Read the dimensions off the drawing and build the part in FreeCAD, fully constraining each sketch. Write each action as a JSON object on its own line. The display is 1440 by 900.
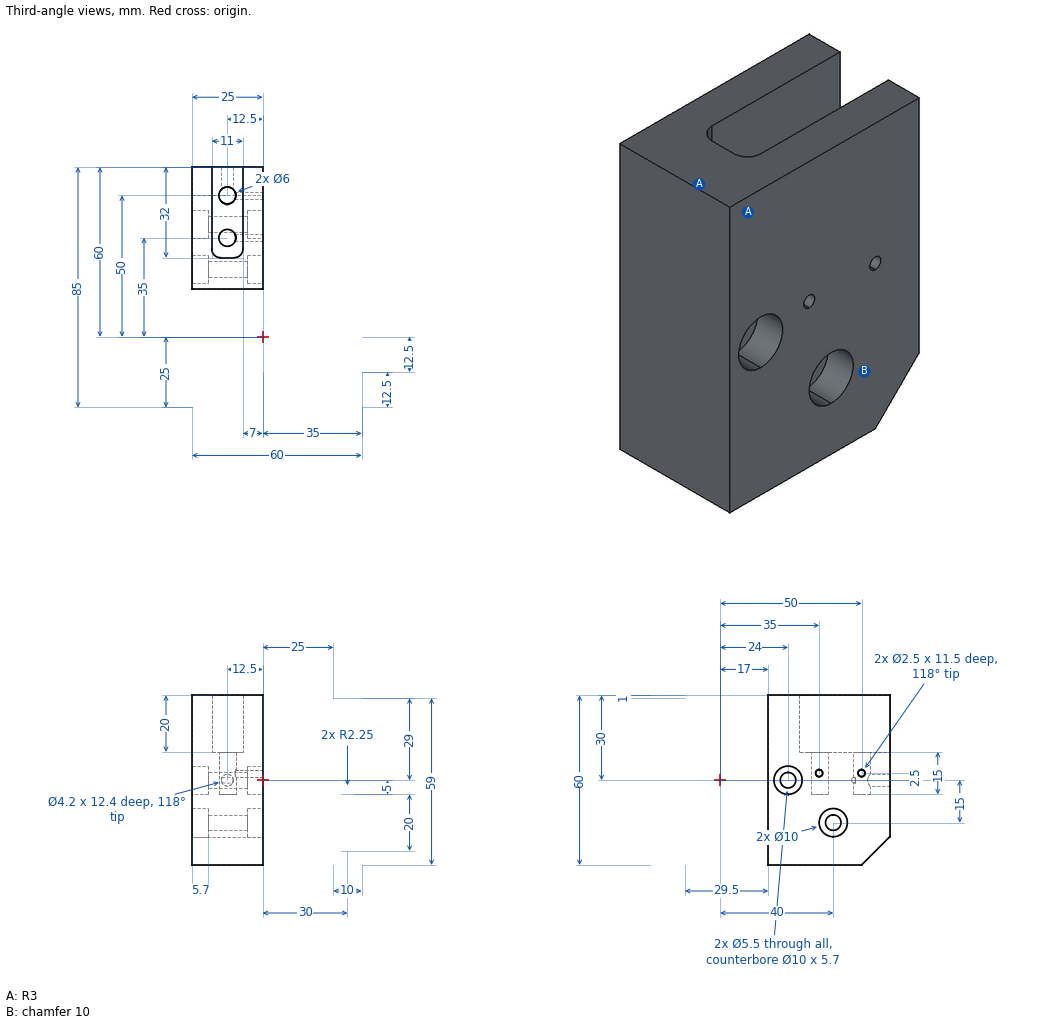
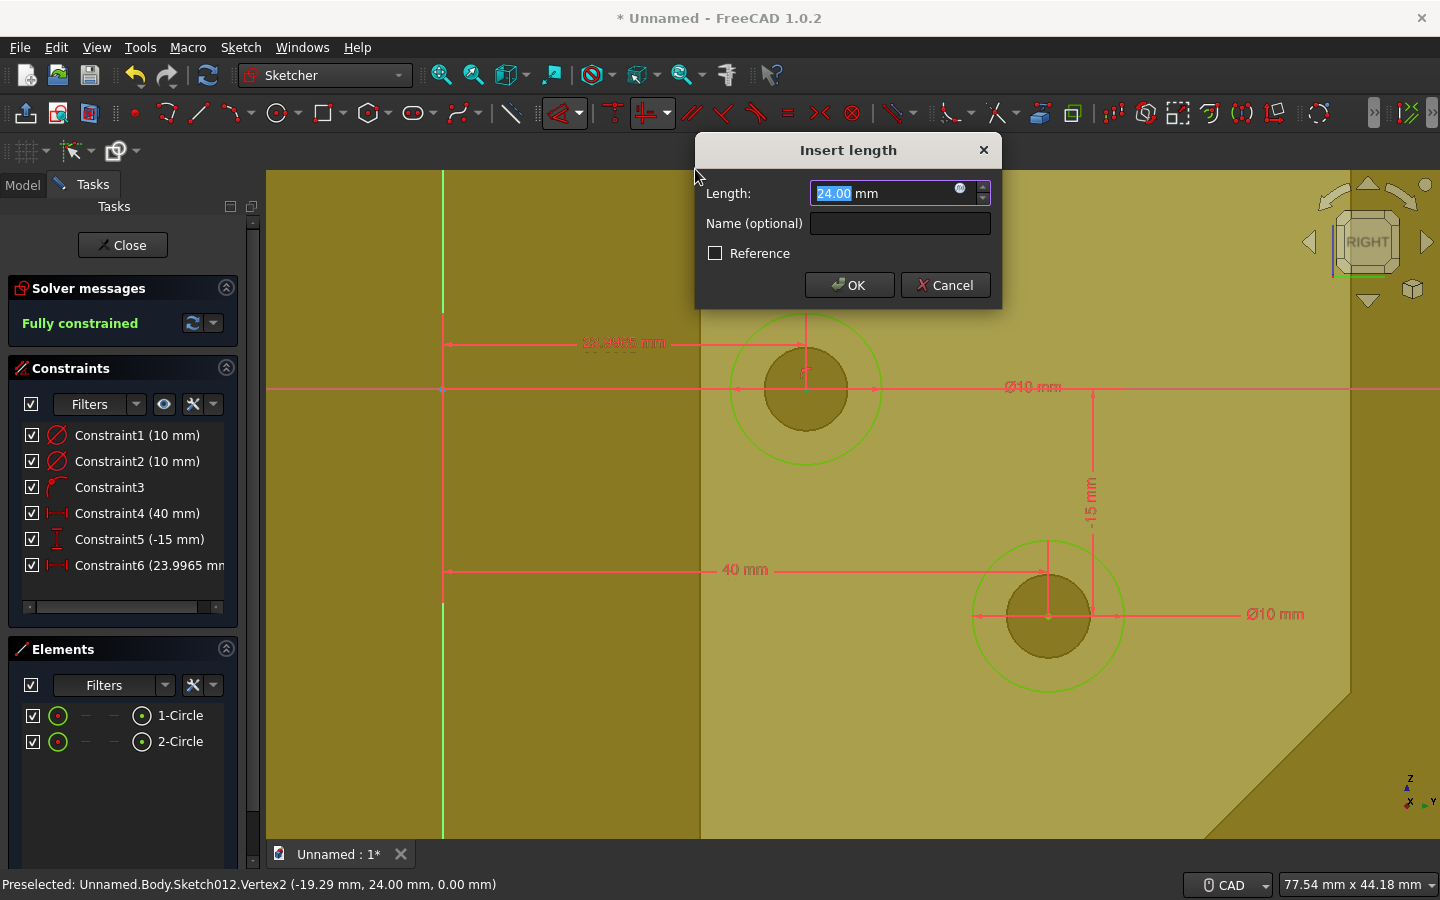
{"action": "type", "text": "24"}
{"action": "key", "text": "Return"}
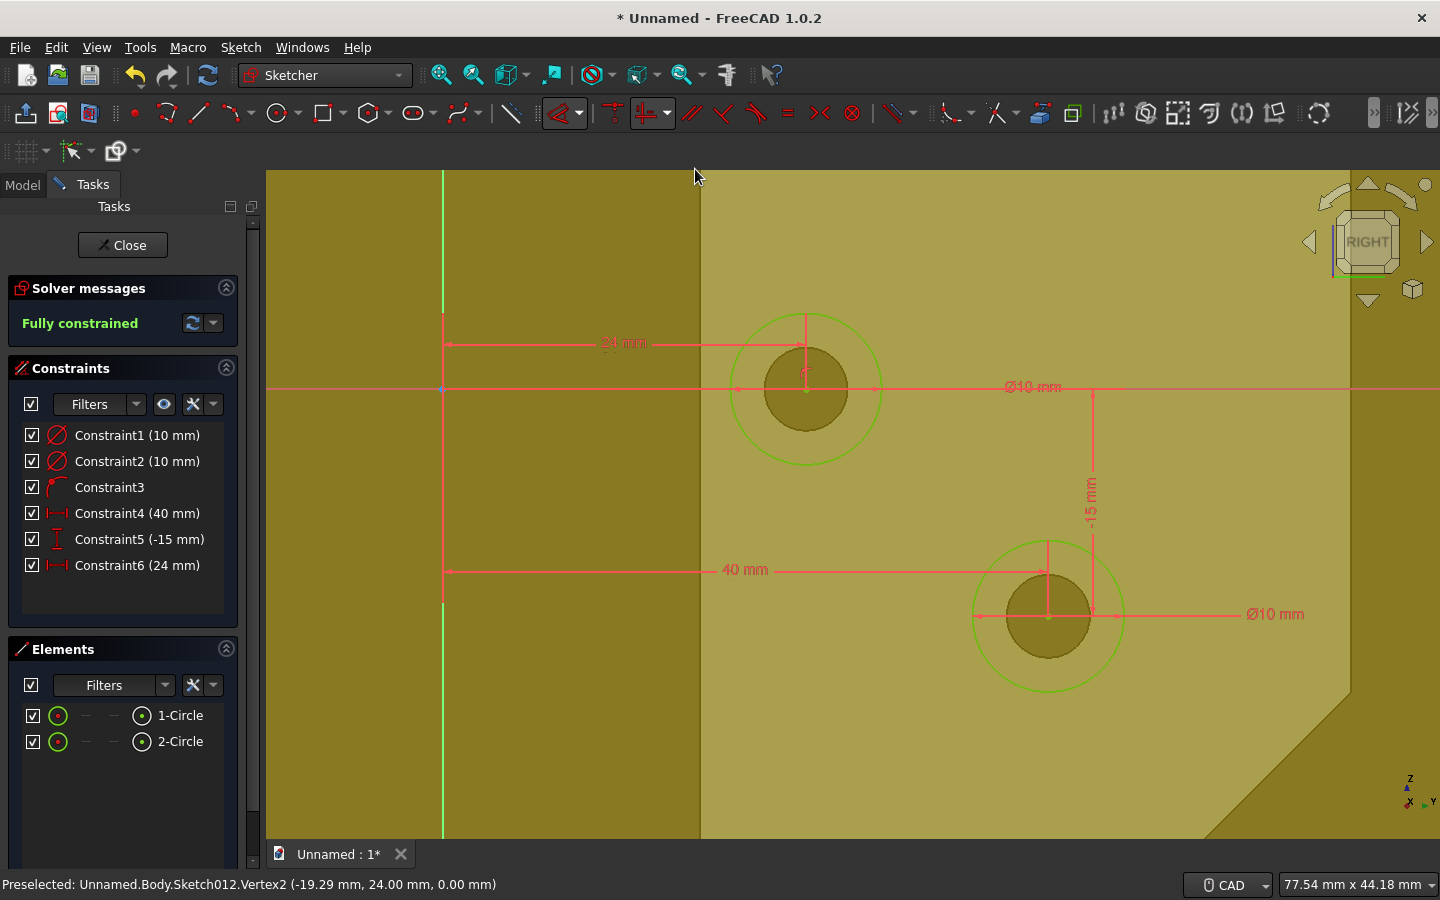
{"action": "left_click", "coordinate": [123, 245]}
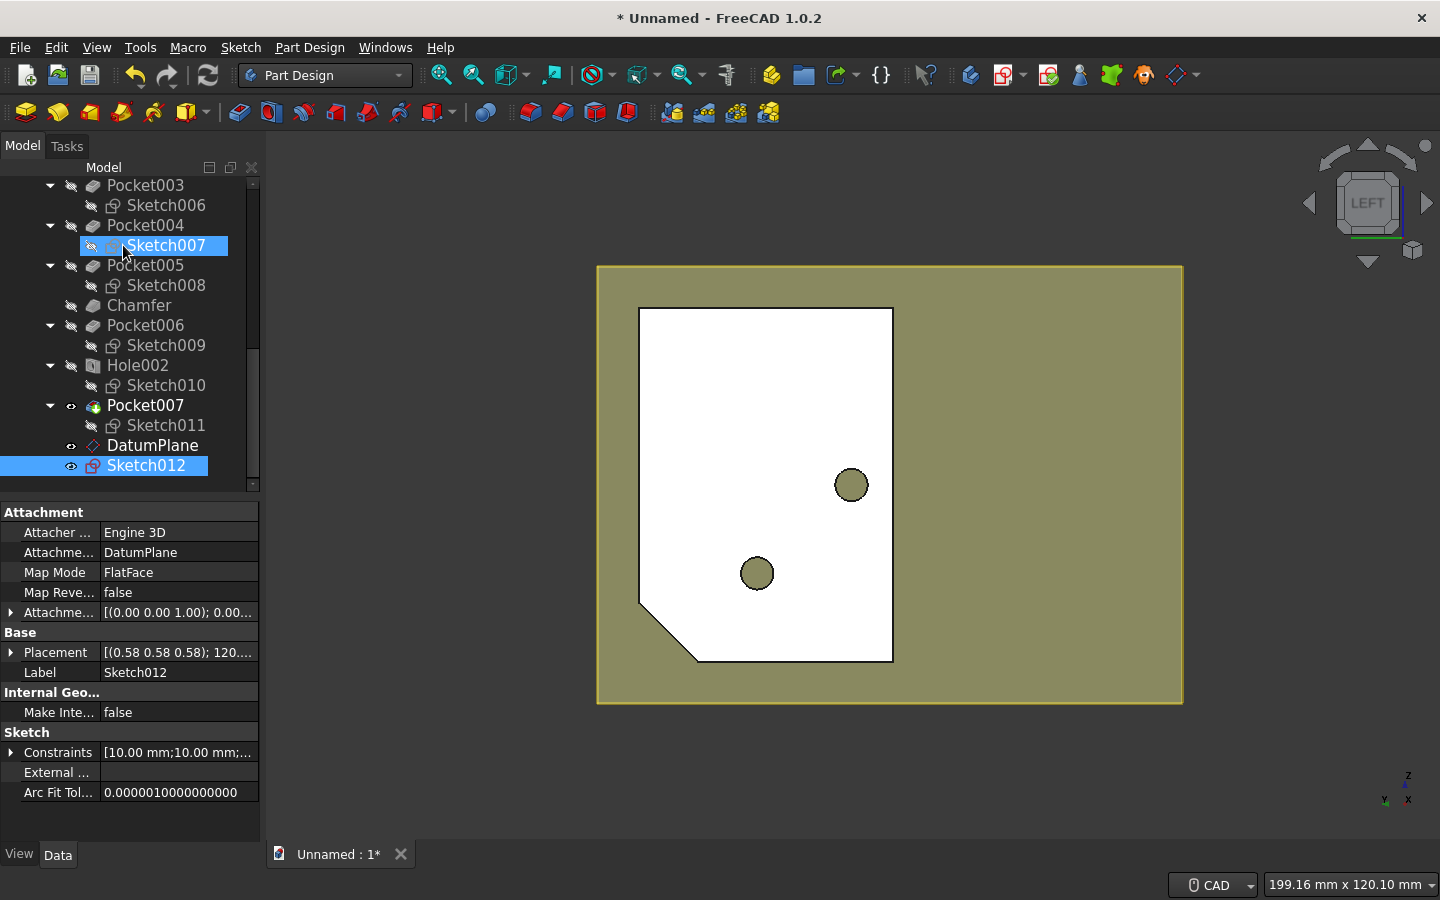
{"action": "left_click", "coordinate": [240, 112]}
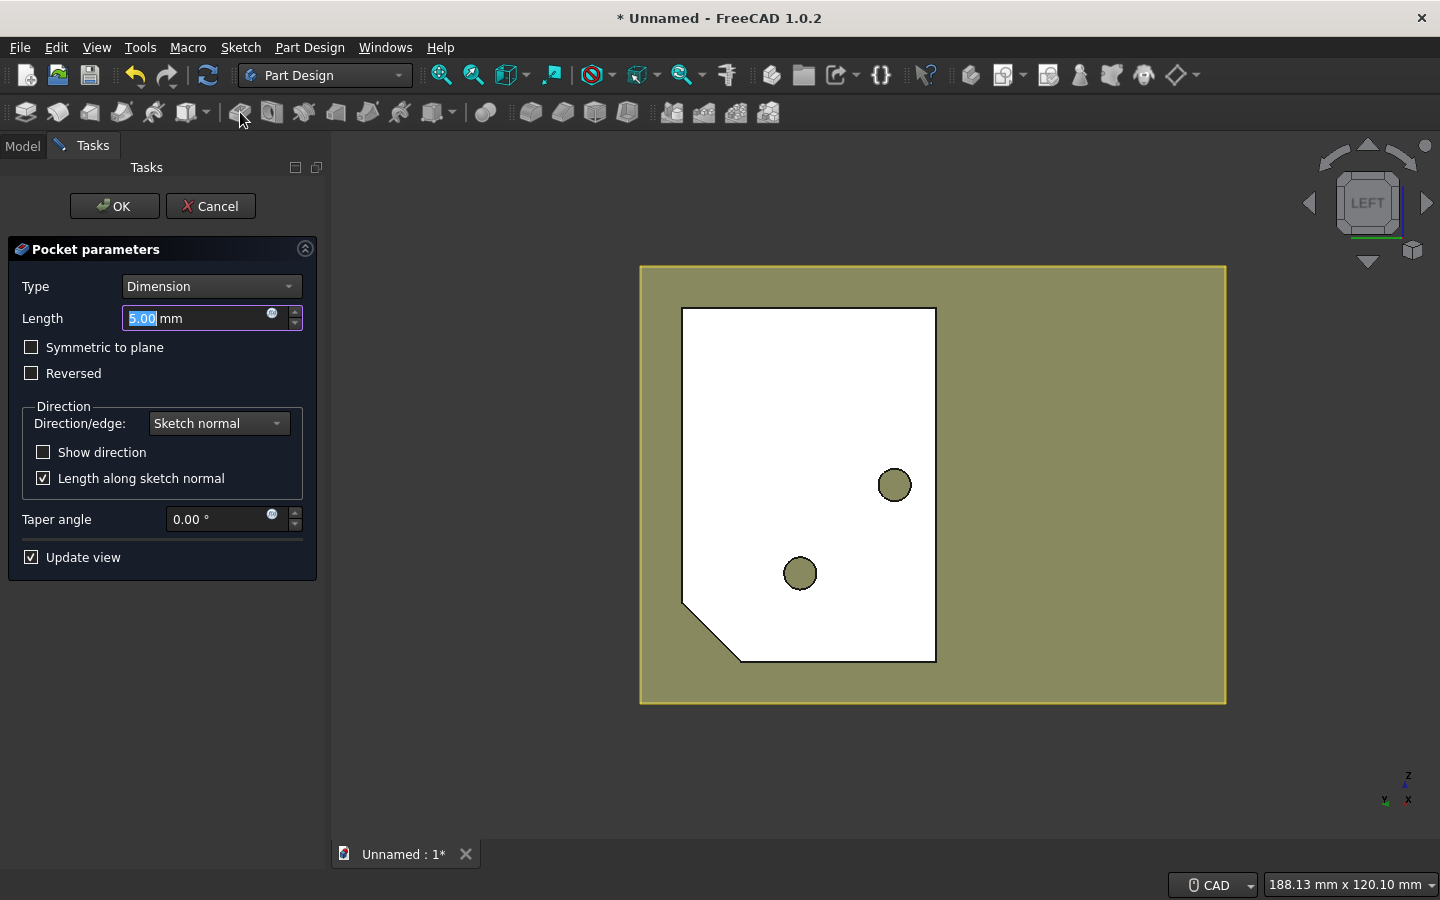
{"action": "type", "text": "5.7"}
{"action": "key", "text": "Tab"}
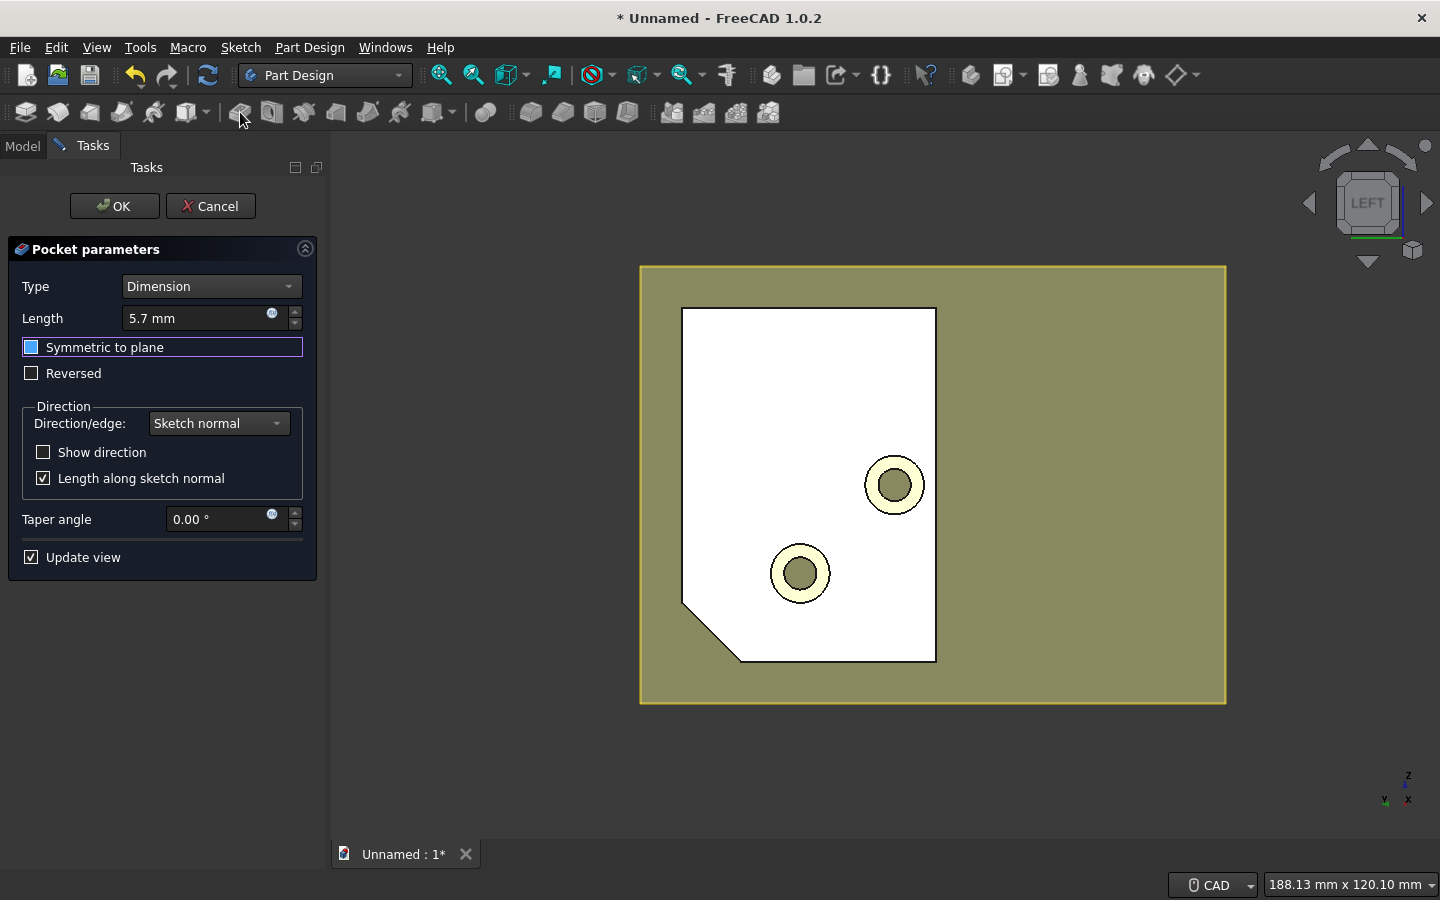
{"action": "left_click", "coordinate": [115, 206]}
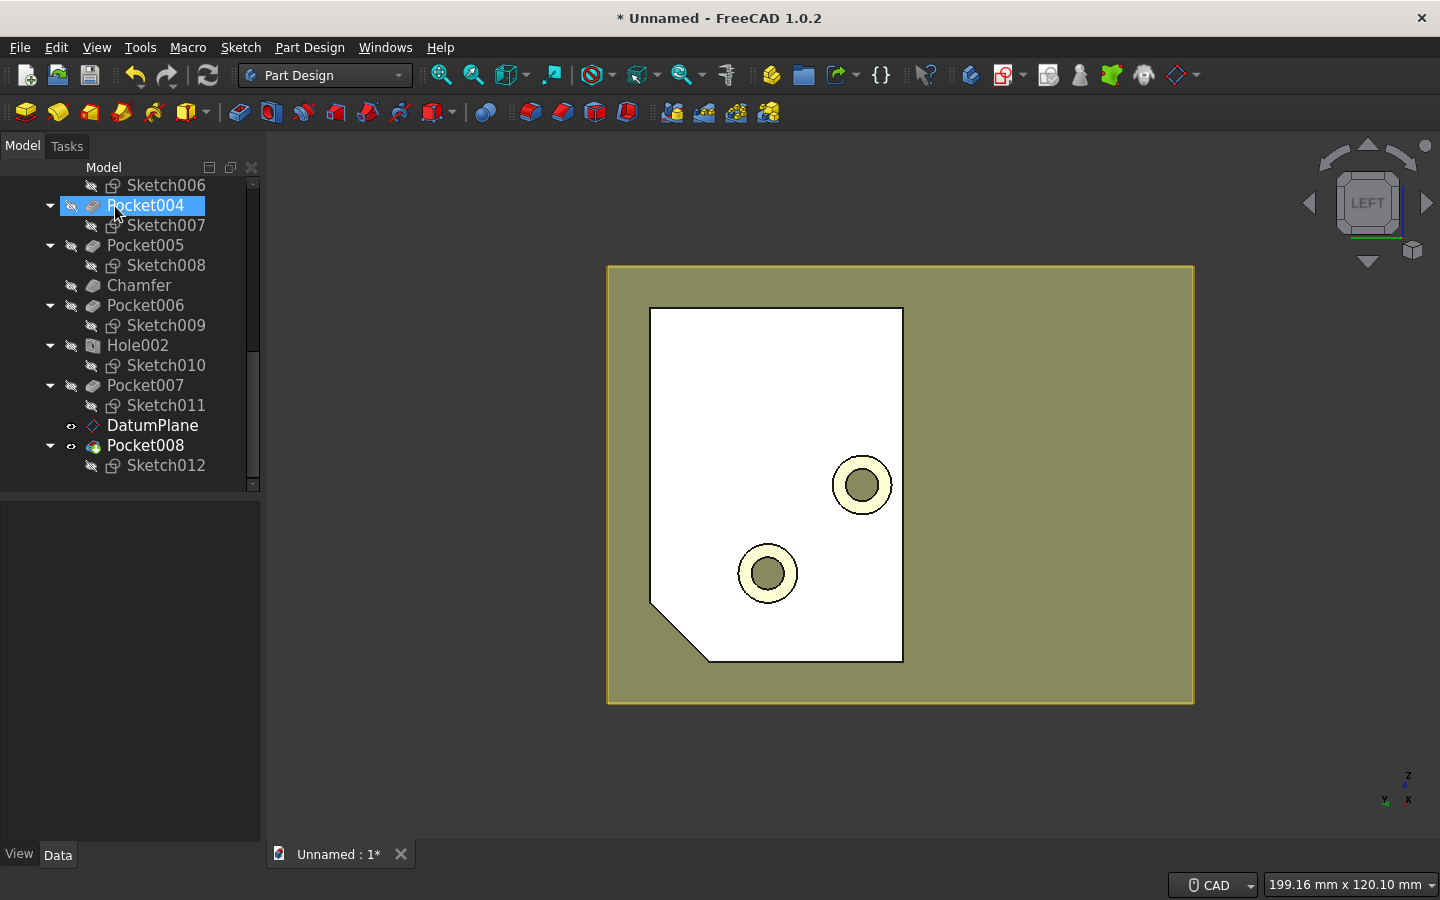
{"action": "left_click", "coordinate": [116, 426]}
{"action": "key", "text": "space"}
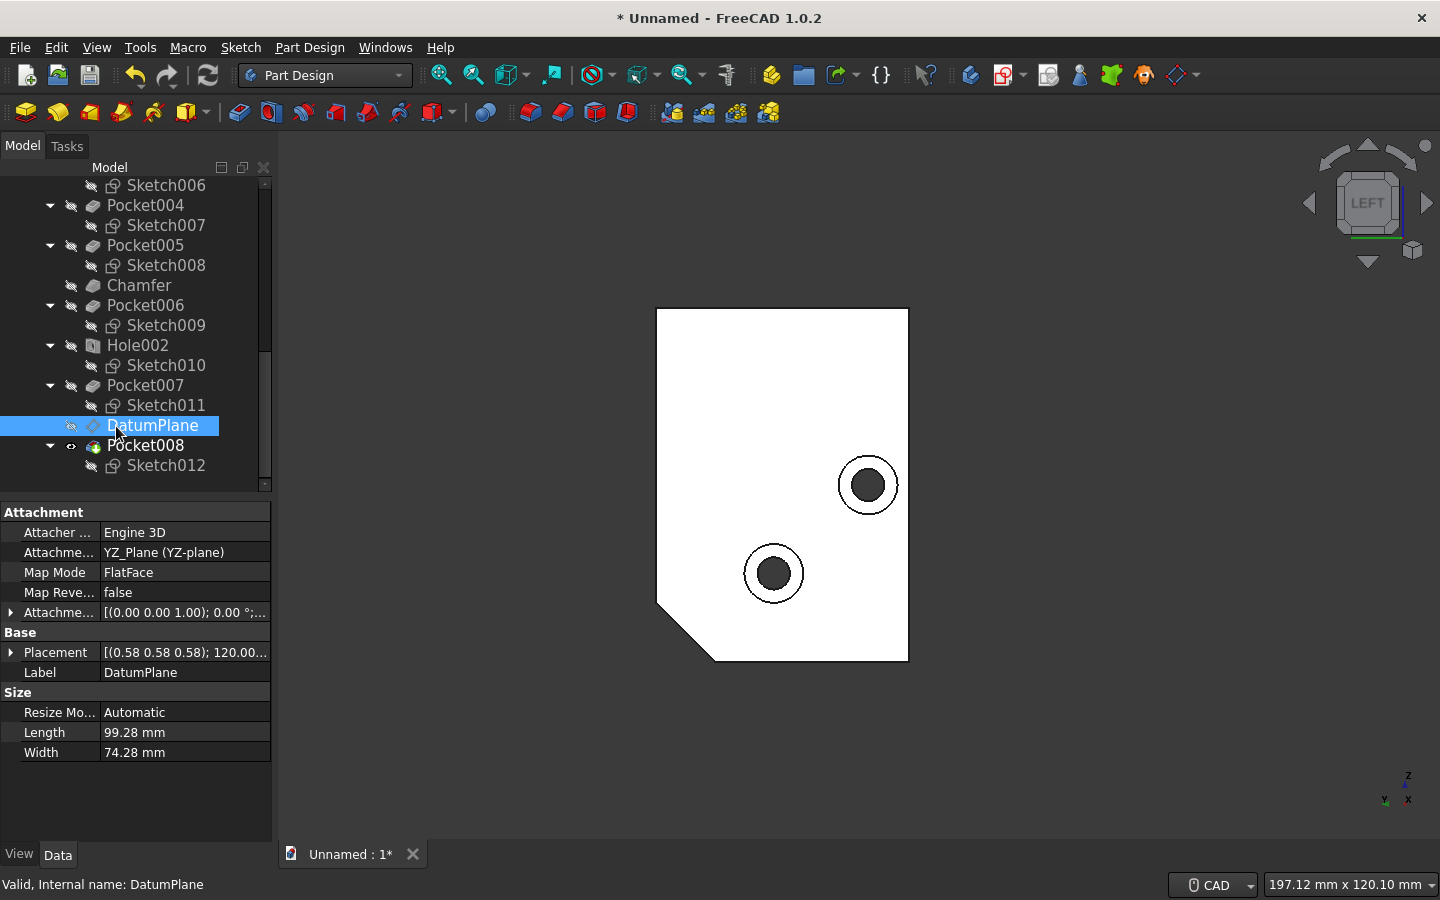
{"action": "key", "text": "0"}